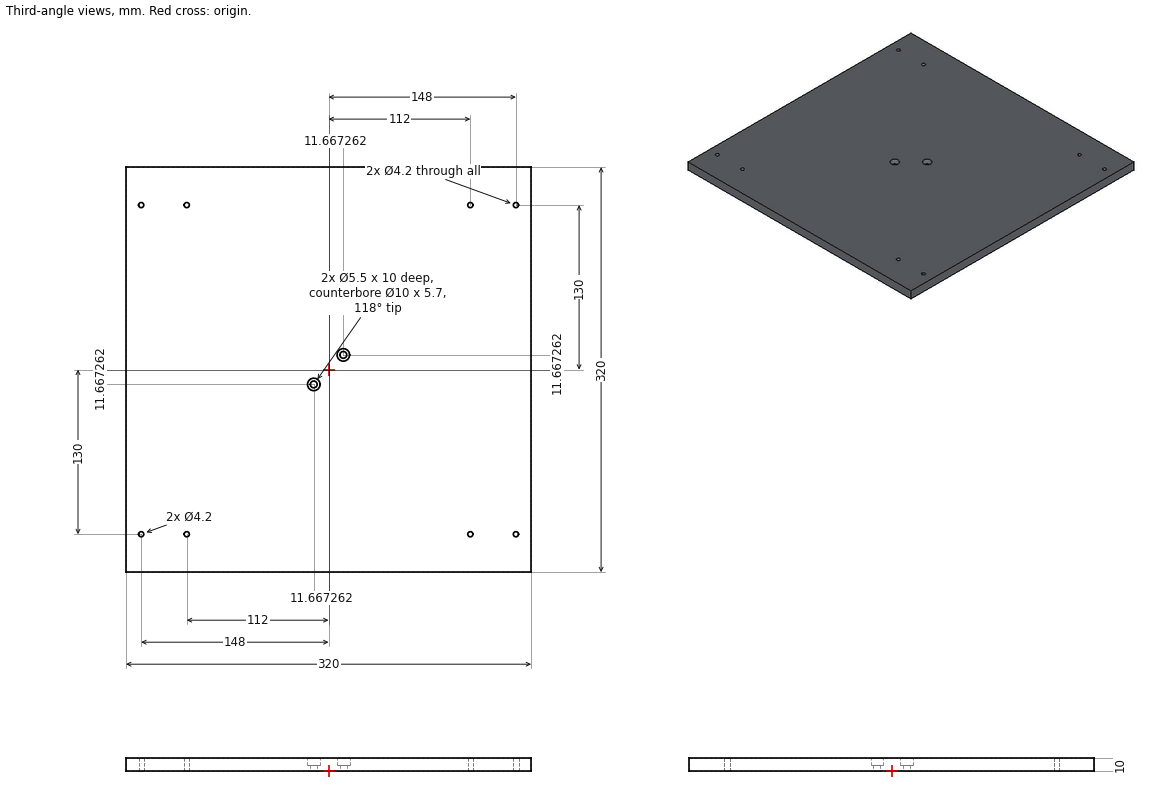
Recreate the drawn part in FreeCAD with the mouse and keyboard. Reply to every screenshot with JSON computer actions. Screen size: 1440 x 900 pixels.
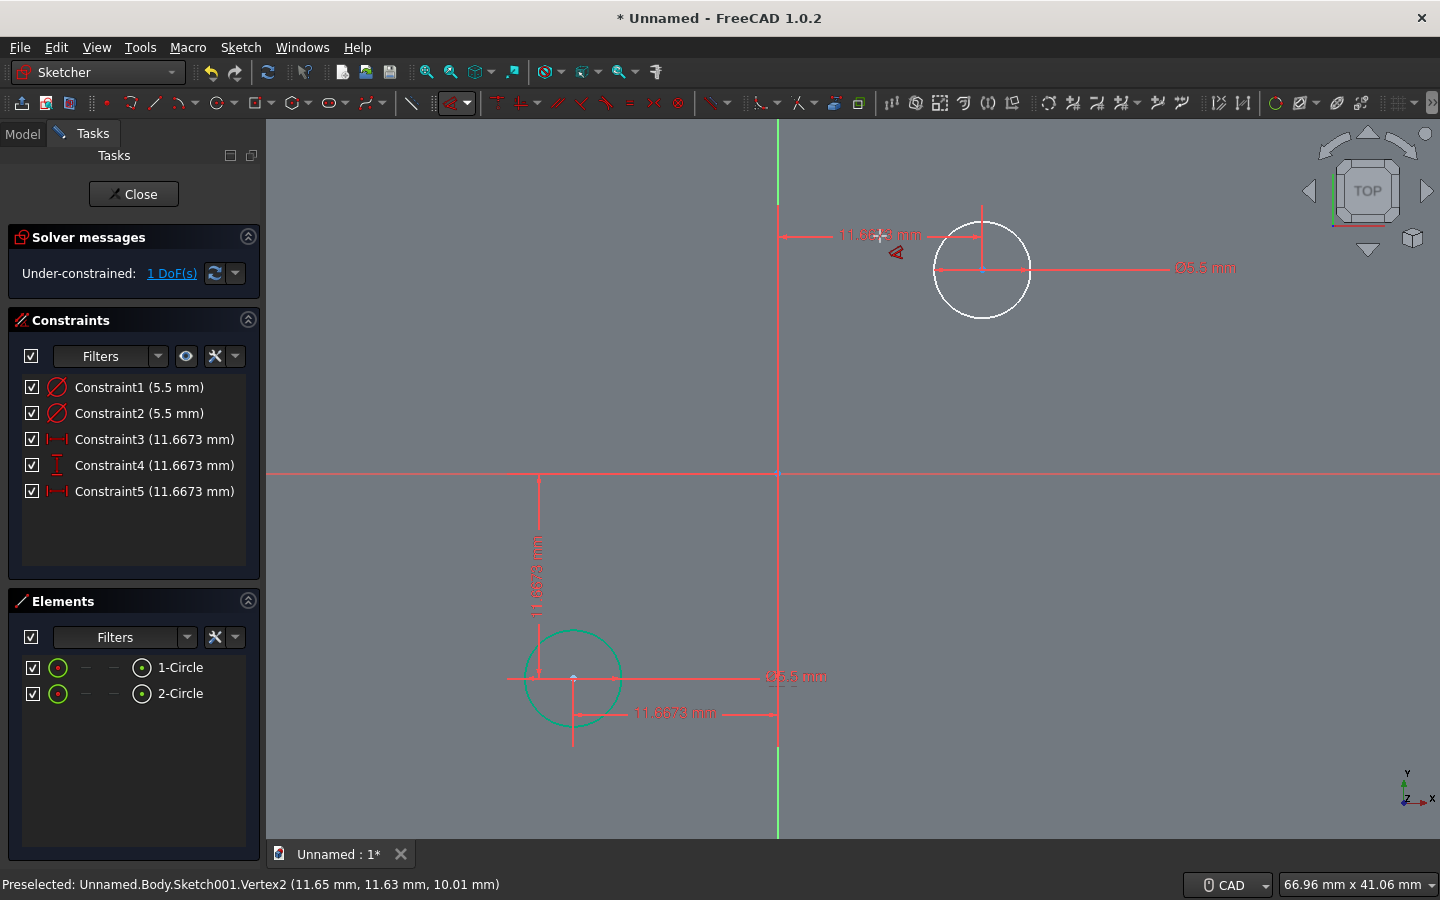
{"action": "left_click", "coordinate": [982, 270]}
{"action": "left_click", "coordinate": [1016, 372]}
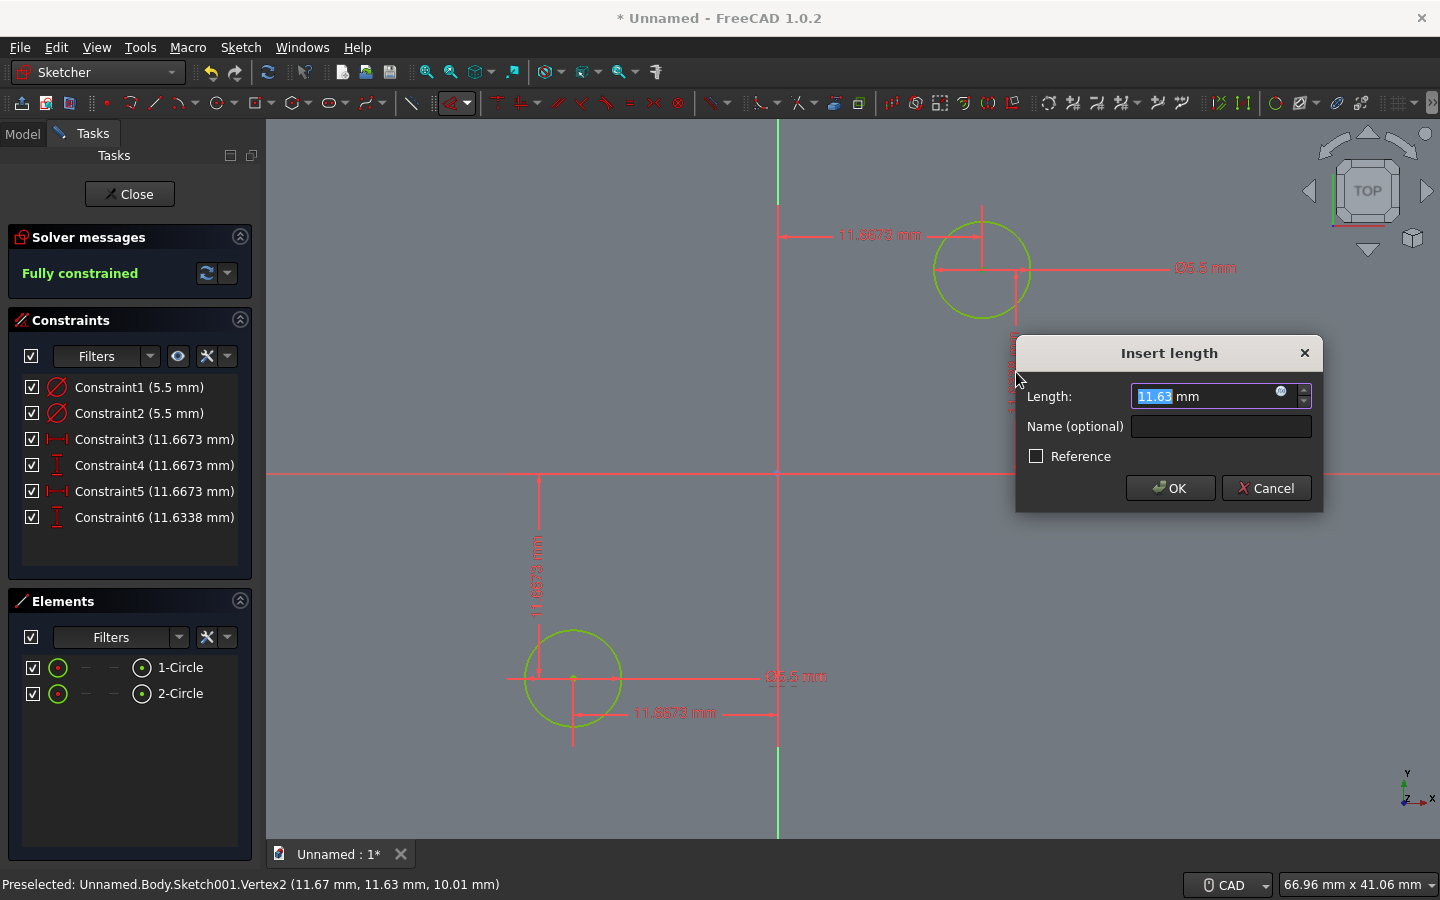
{"action": "type", "text": "11.667262"}
{"action": "key", "text": "Return"}
{"action": "key", "text": "Escape"}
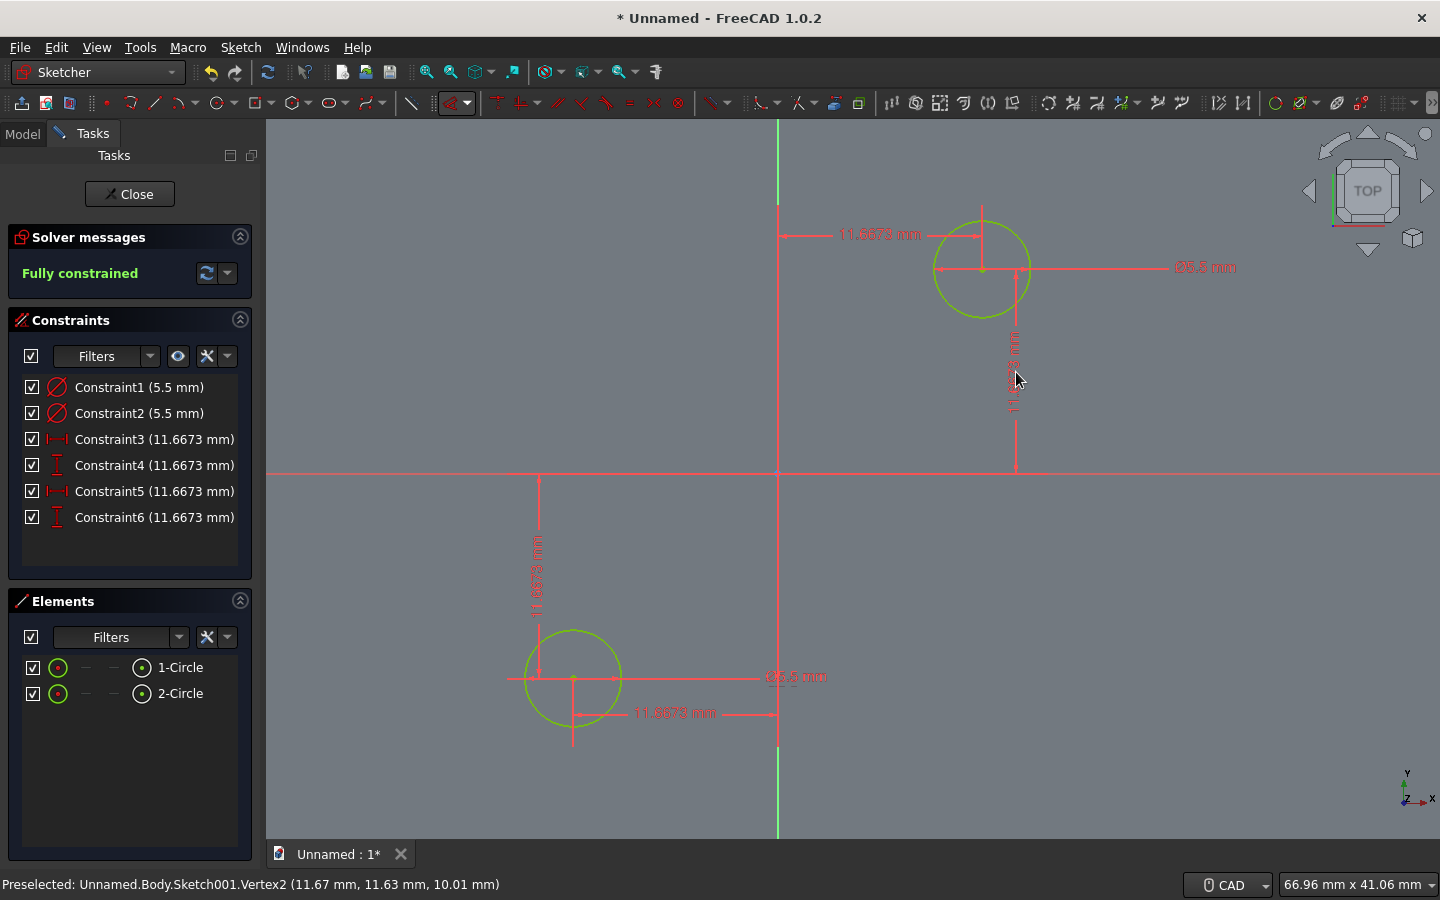
{"action": "left_click", "coordinate": [130, 194]}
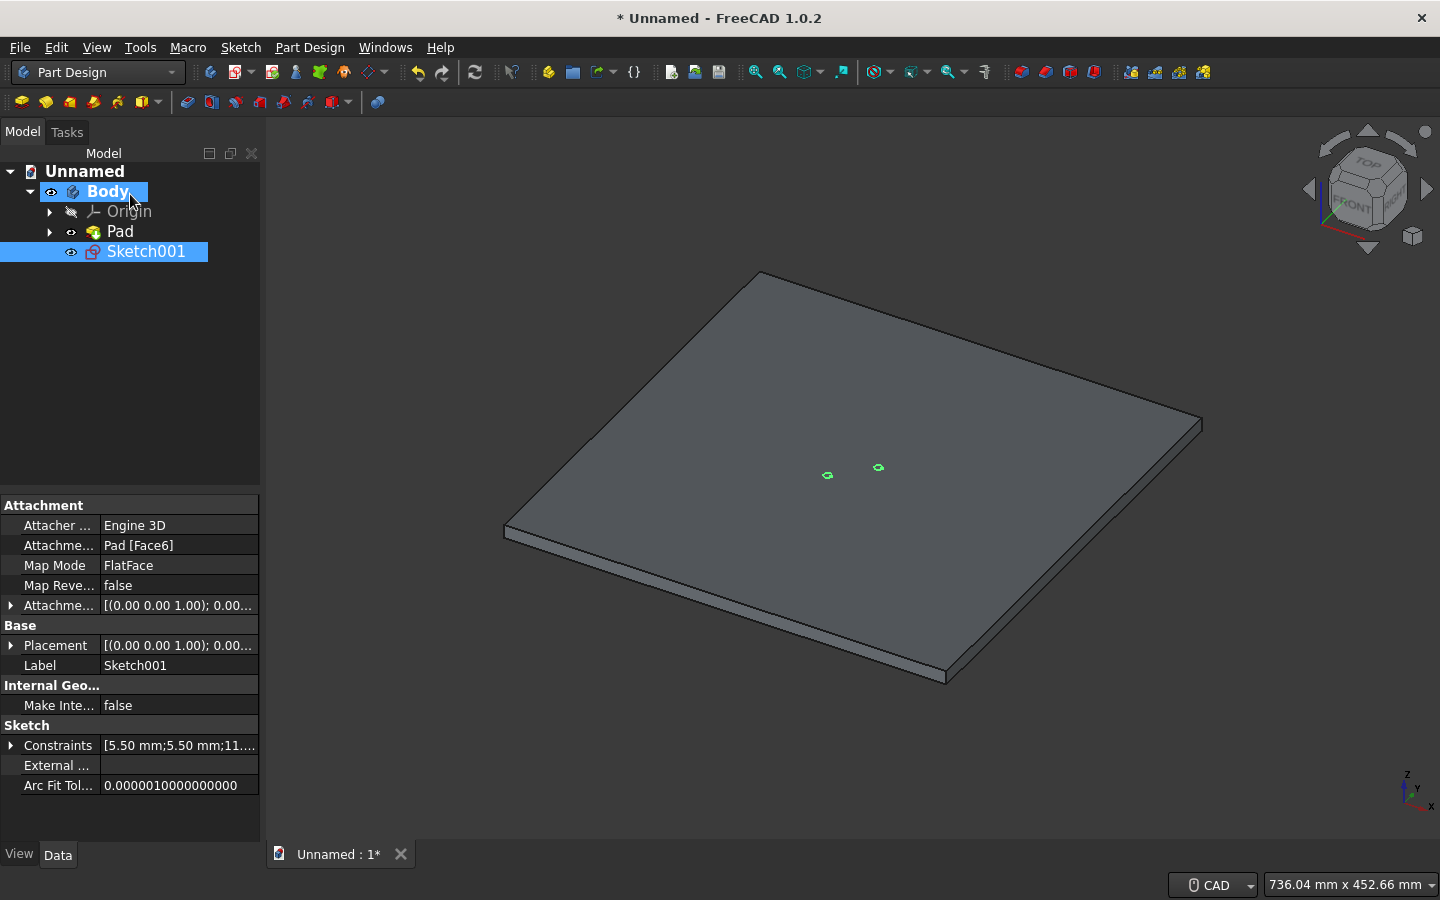
{"action": "left_click", "coordinate": [212, 102]}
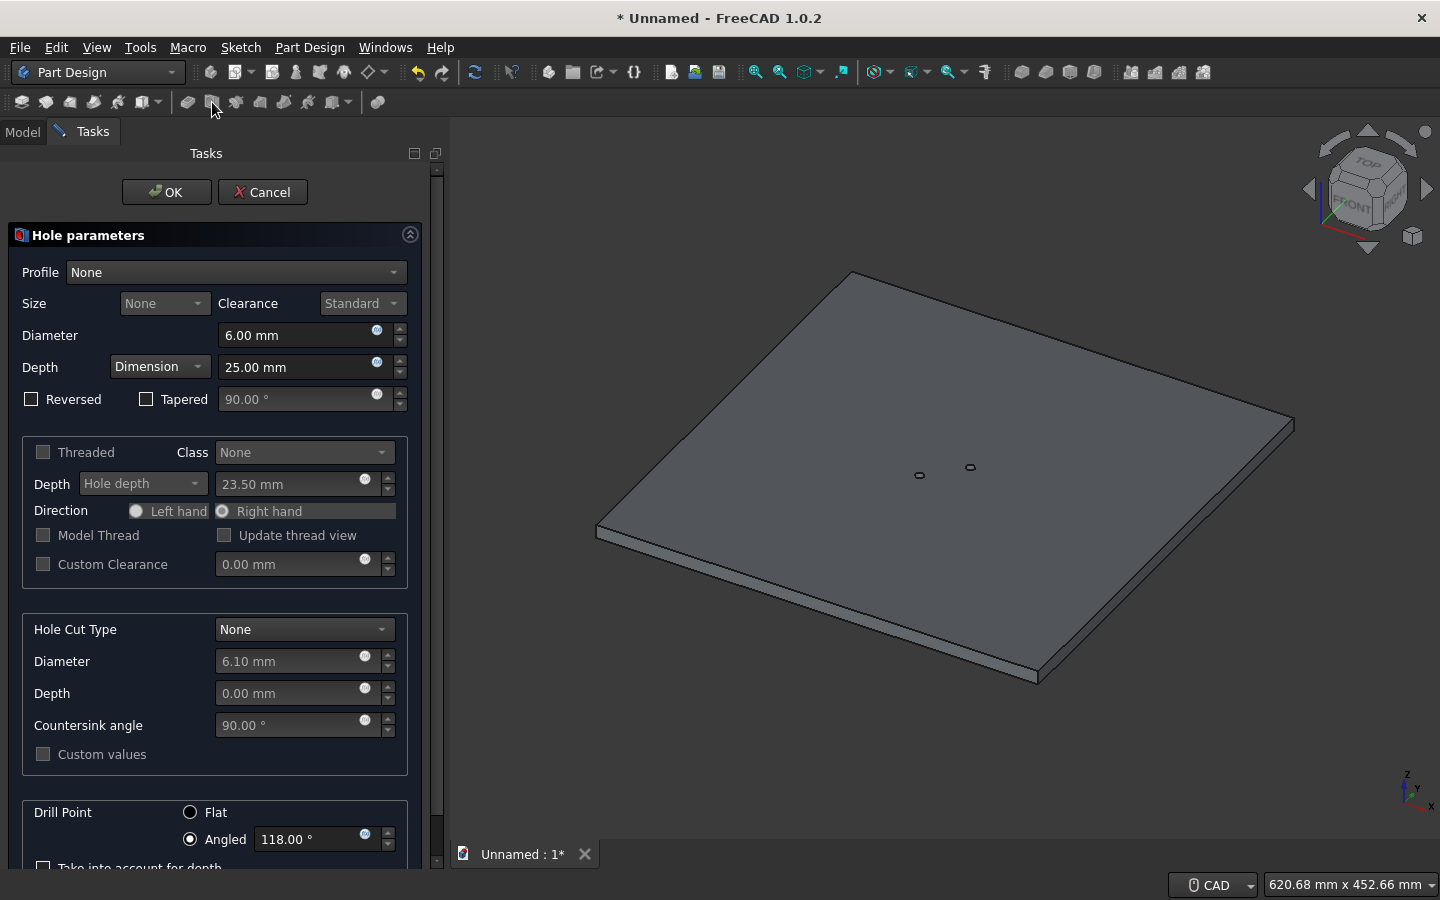
{"action": "triple_click", "coordinate": [305, 335]}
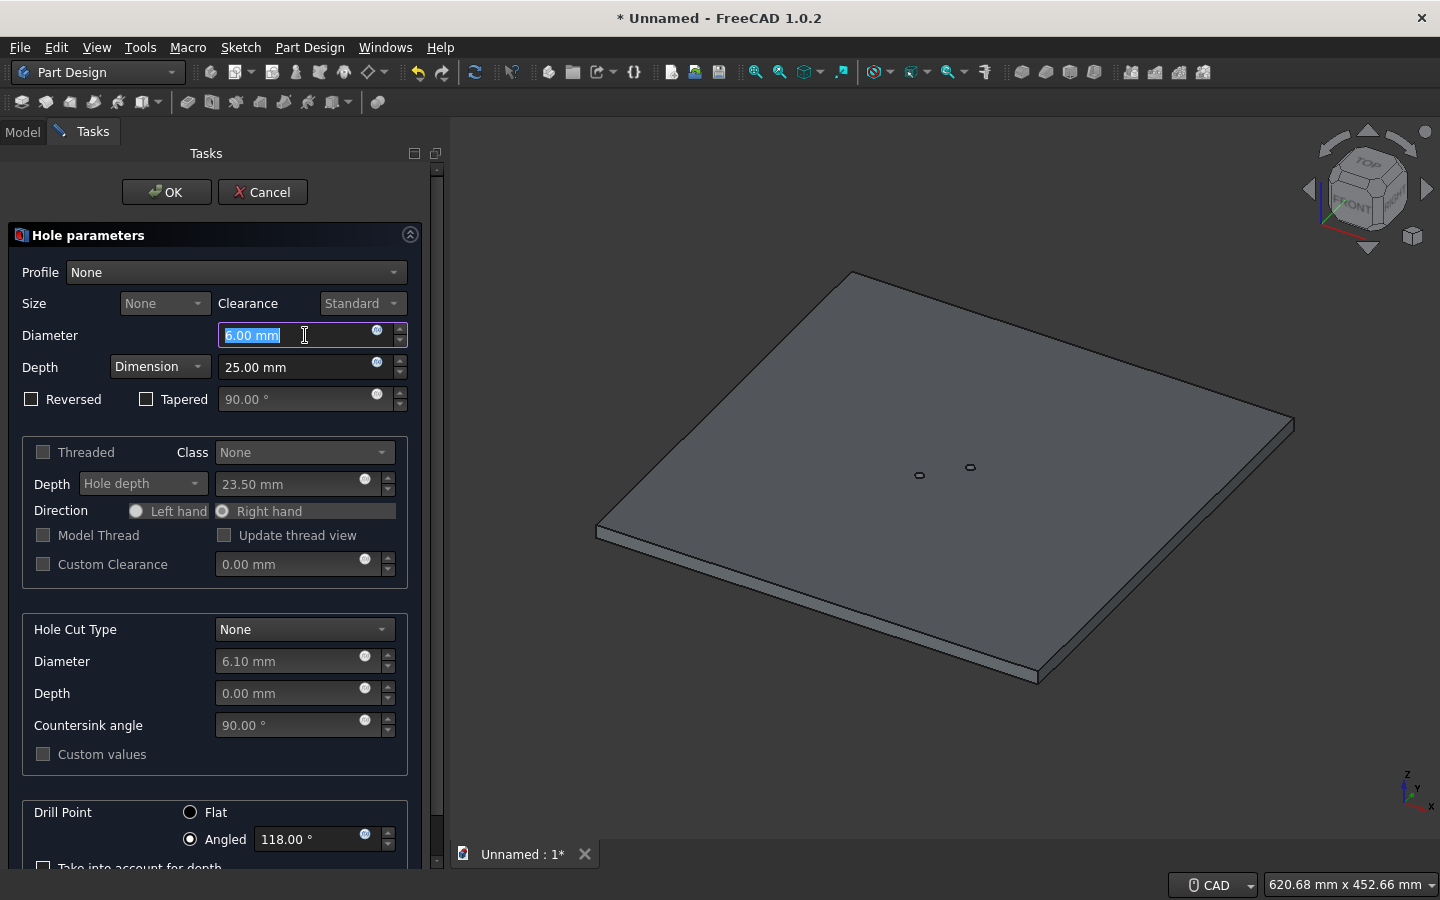
{"action": "type", "text": "5.5"}
{"action": "key", "text": "Tab"}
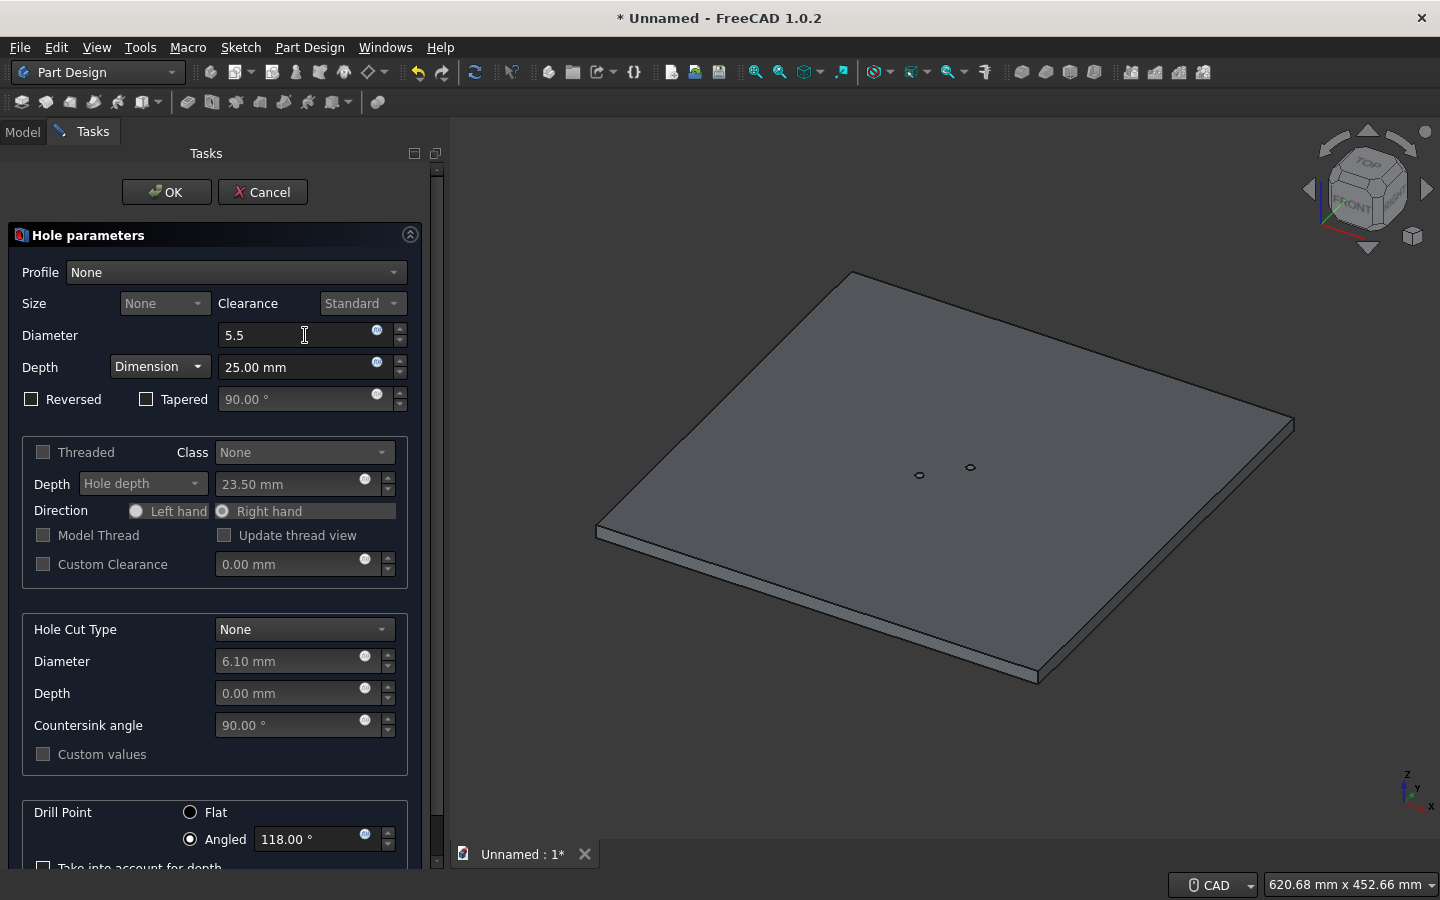
{"action": "triple_click", "coordinate": [305, 367]}